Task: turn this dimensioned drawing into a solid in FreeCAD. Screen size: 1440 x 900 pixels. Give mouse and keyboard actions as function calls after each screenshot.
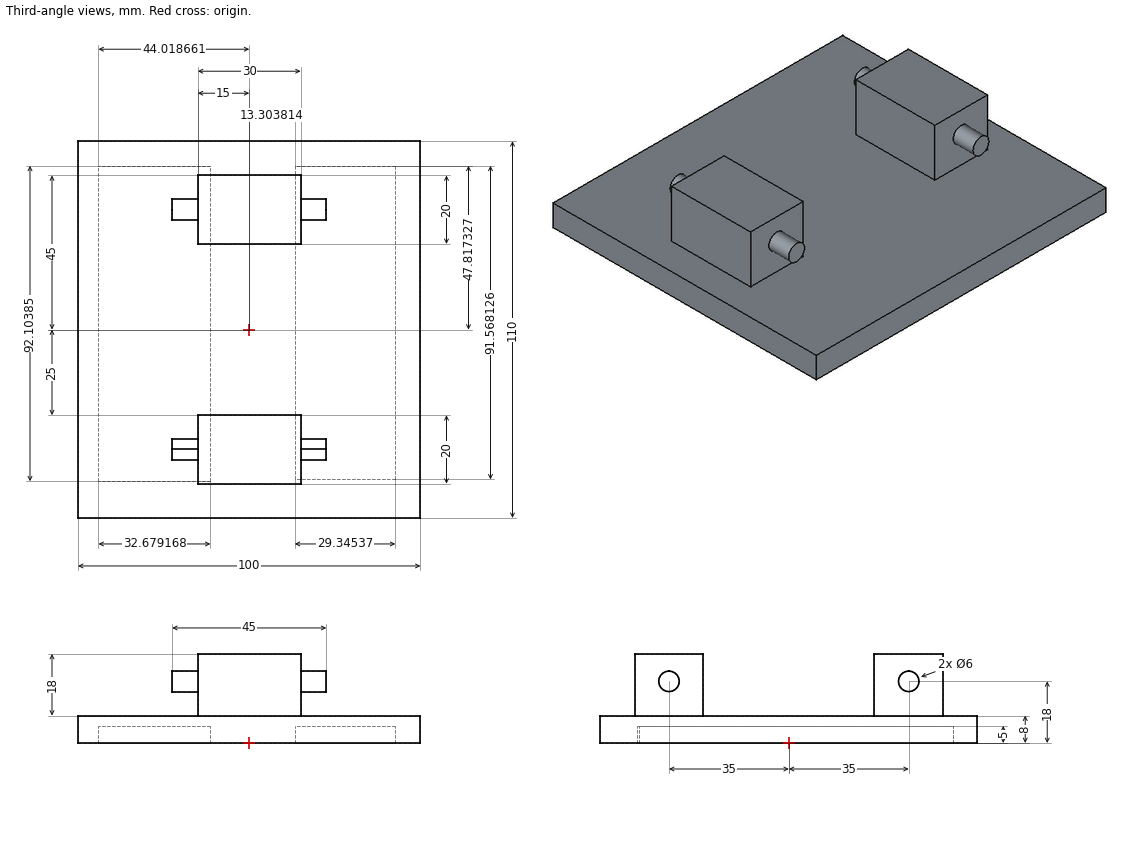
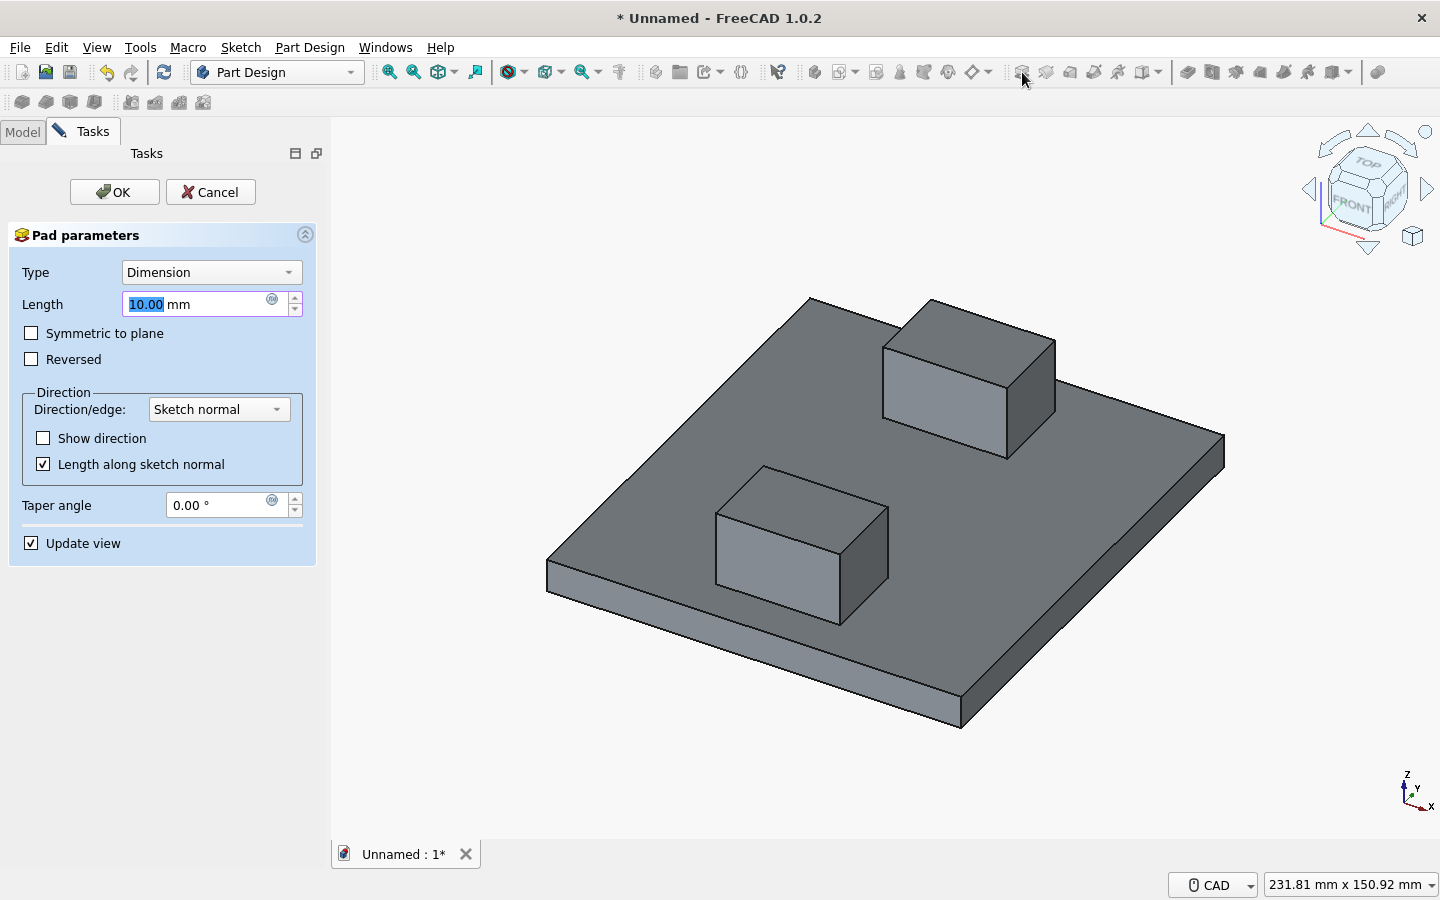
text(45)
key(Tab)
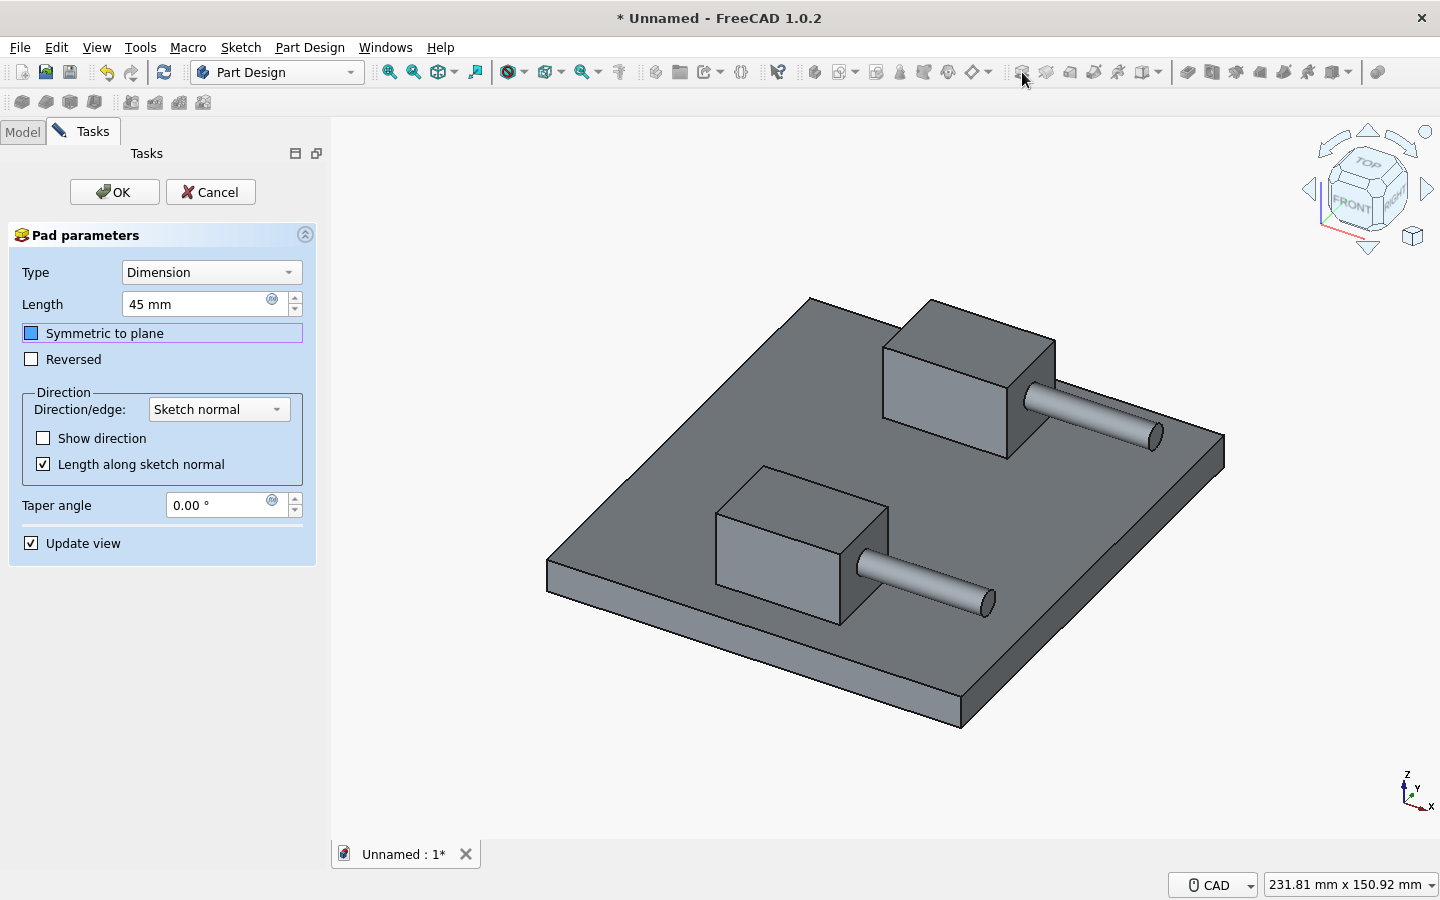
click(30, 333)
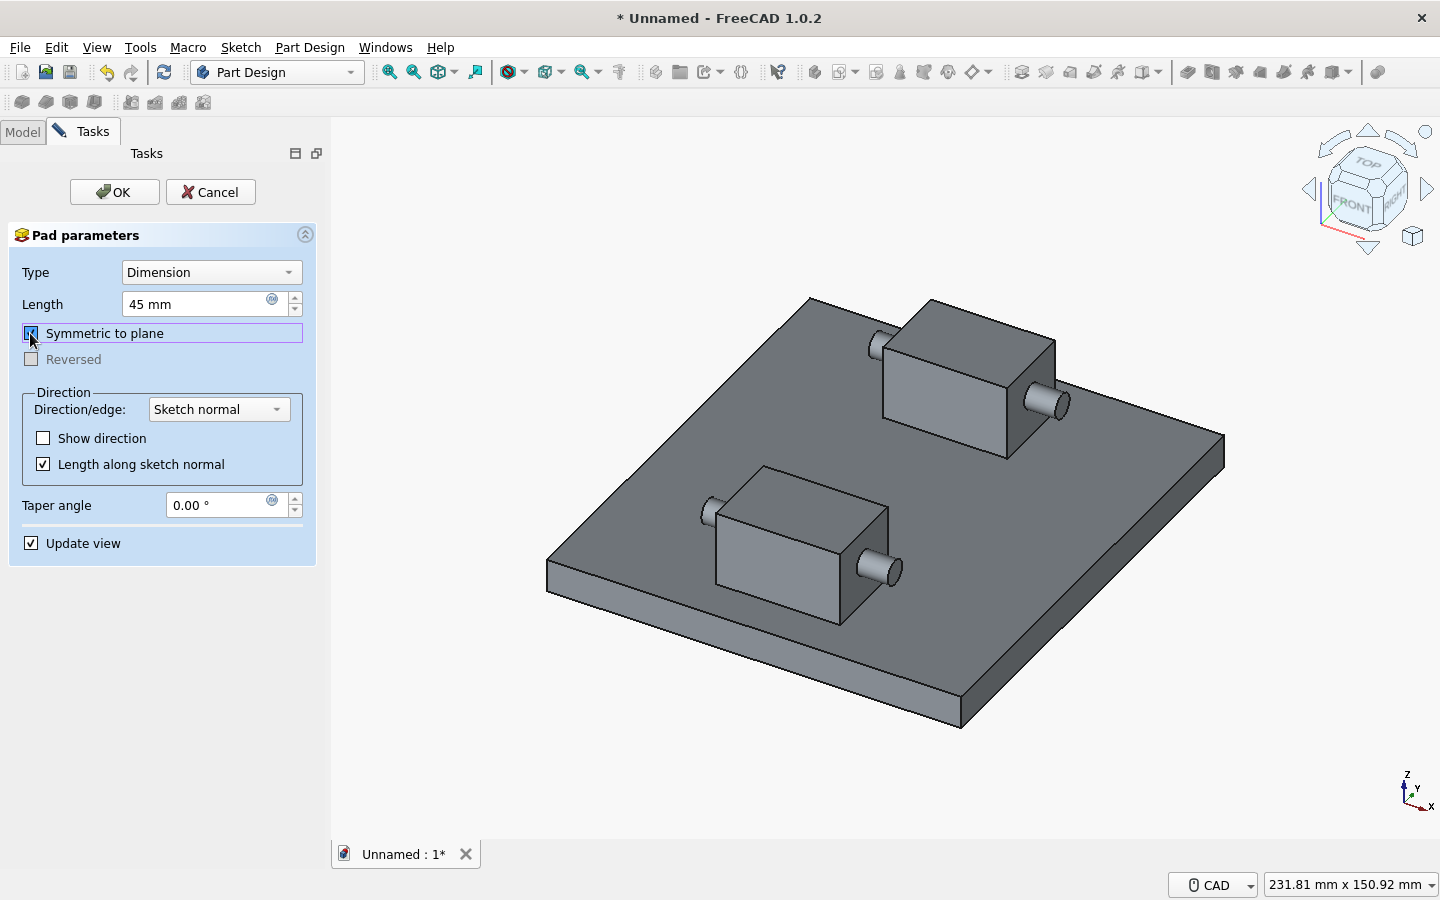
click(115, 192)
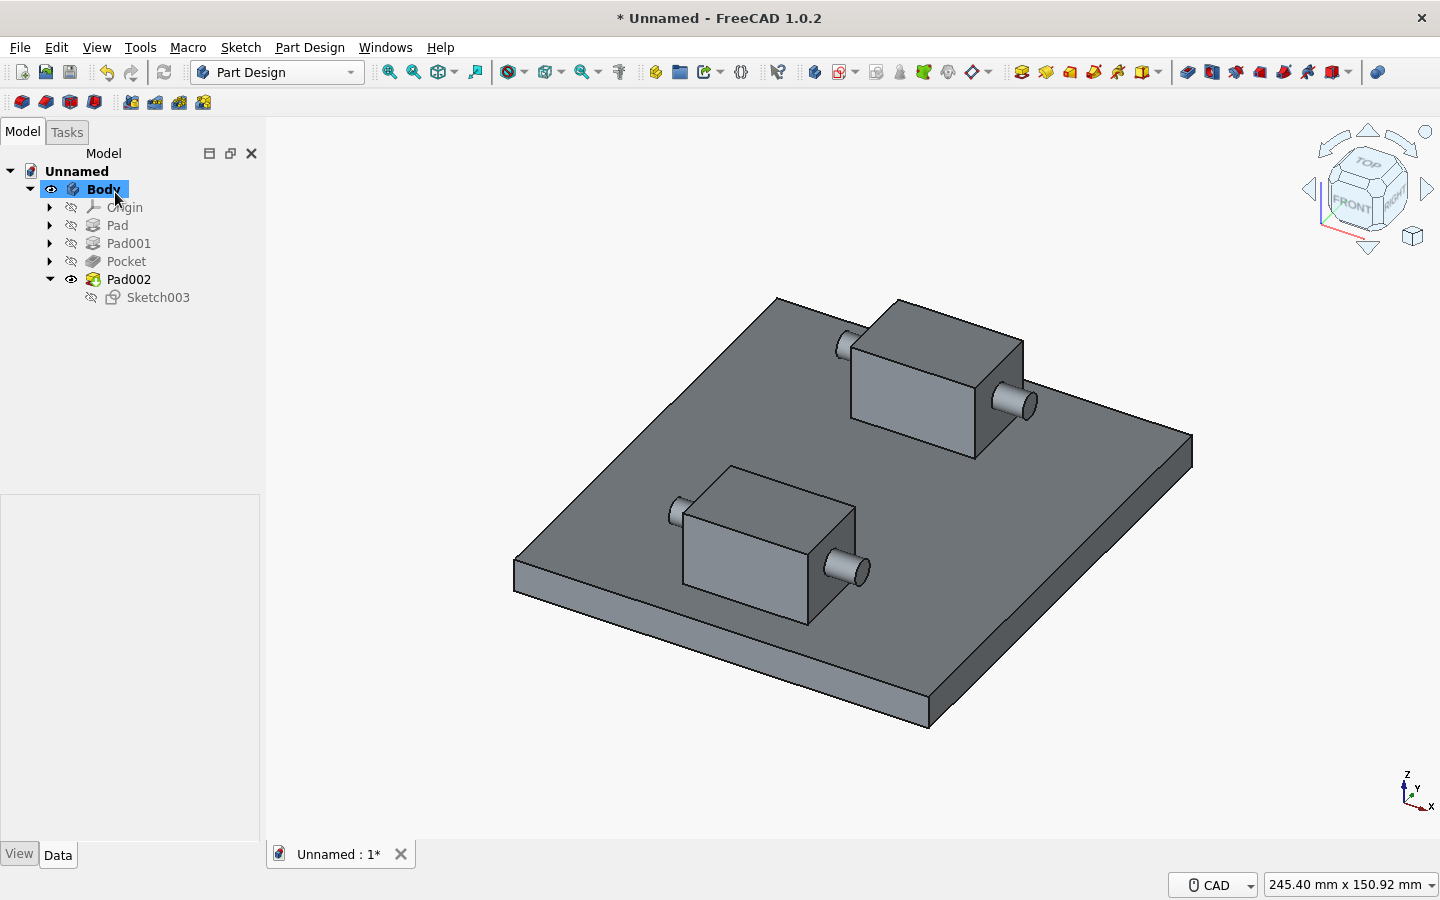
key(0)